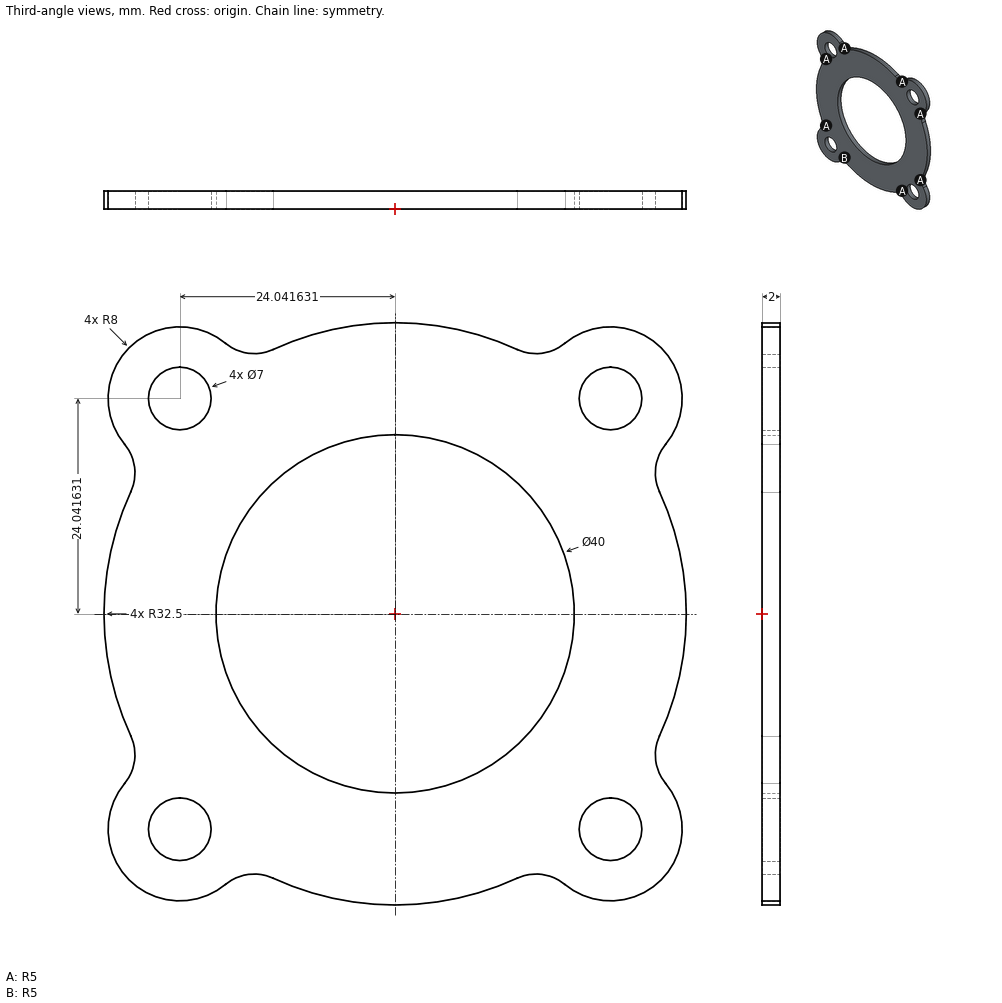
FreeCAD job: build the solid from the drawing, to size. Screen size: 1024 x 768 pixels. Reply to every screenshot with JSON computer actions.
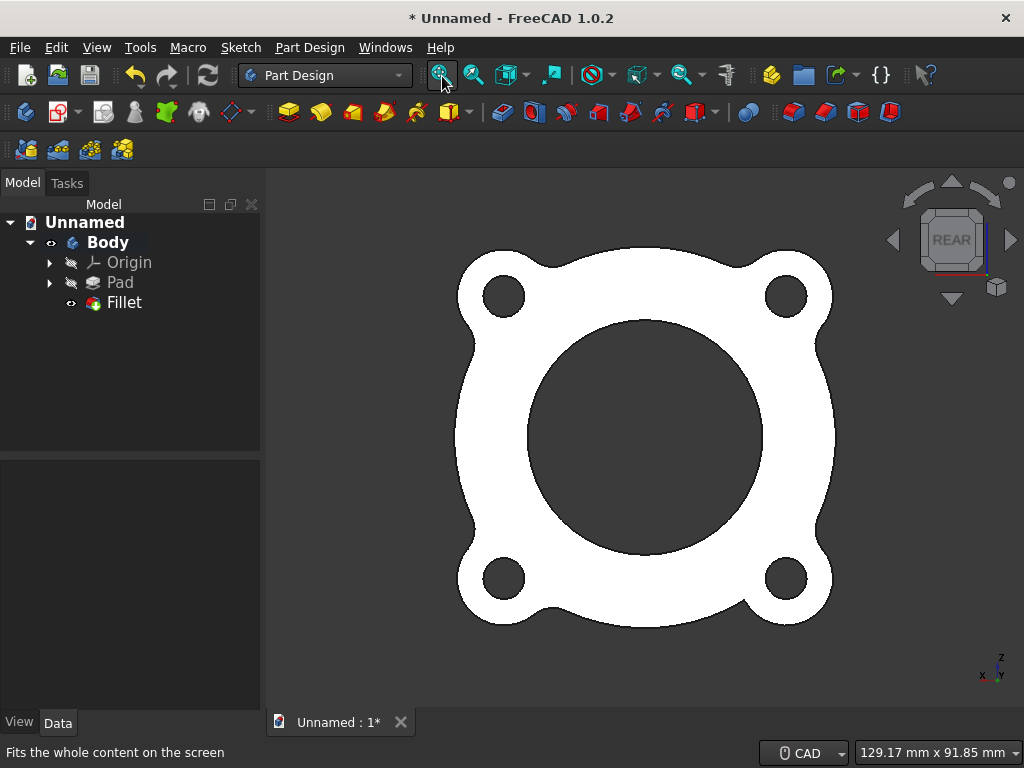
{"action": "scroll", "coordinate": [744, 599], "scroll_direction": "up", "scroll_amount": 7}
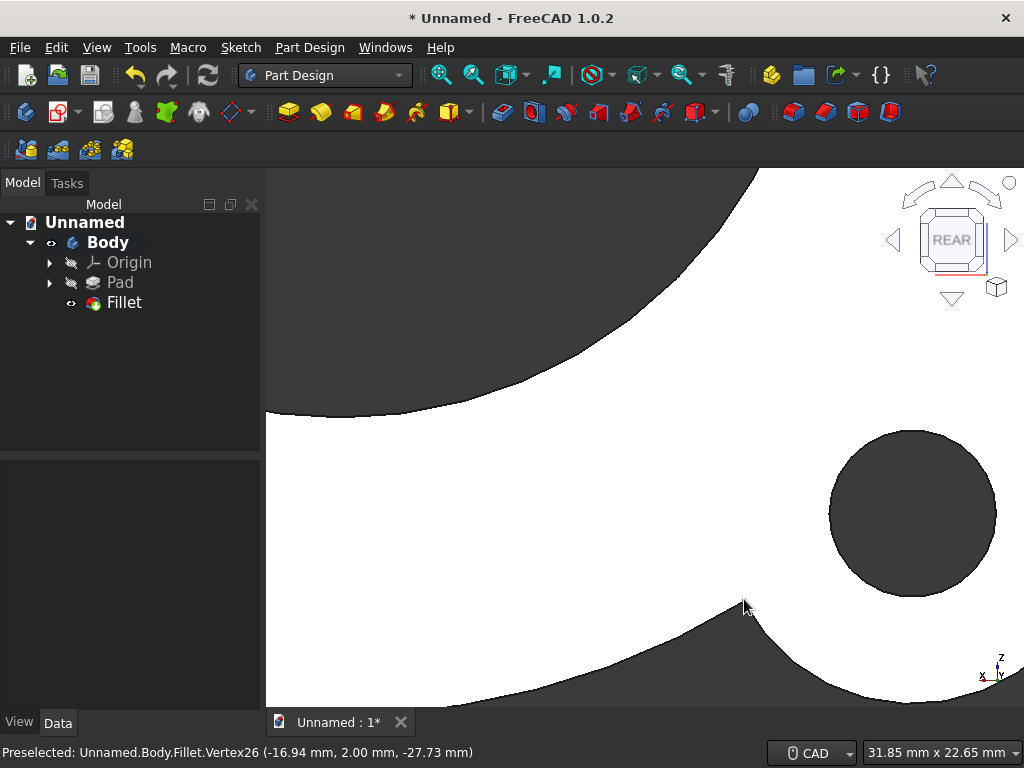
{"action": "left_click", "coordinate": [442, 76]}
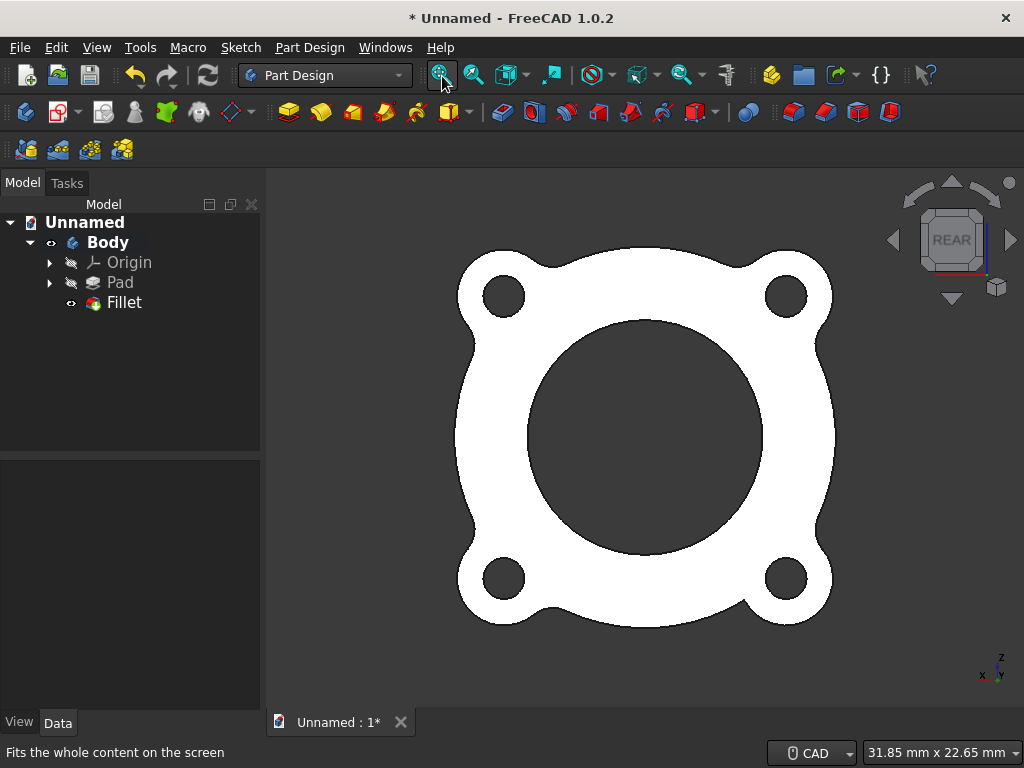
{"action": "key", "text": "6"}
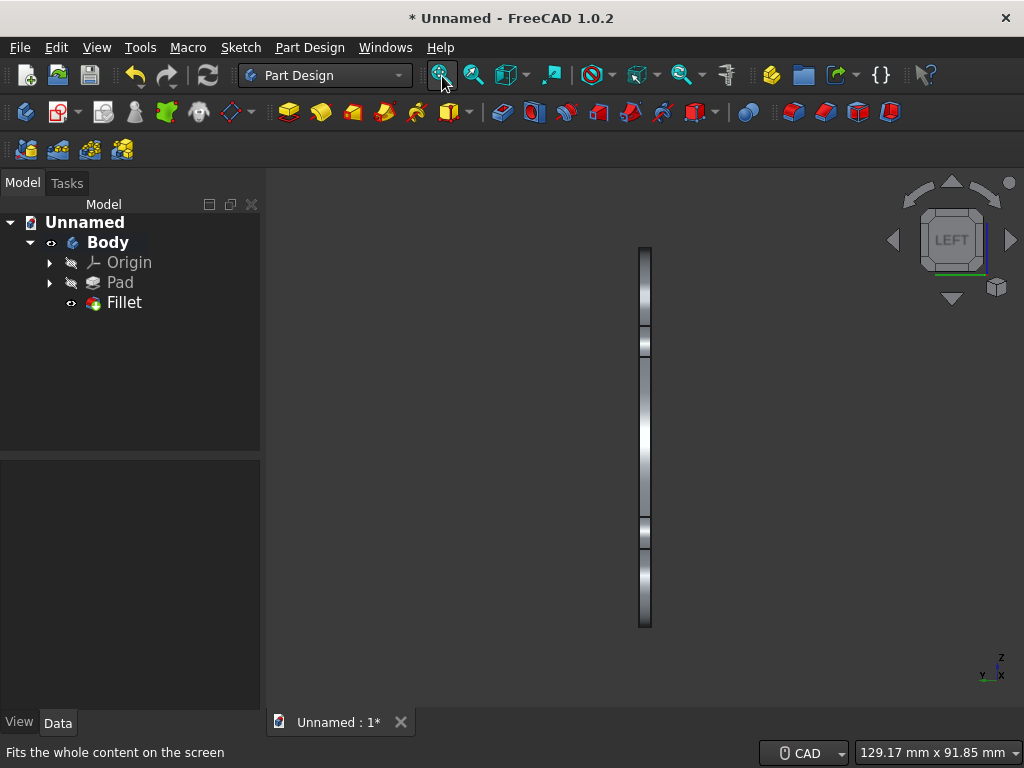
{"action": "scroll", "coordinate": [645, 599], "scroll_direction": "up", "scroll_amount": 7}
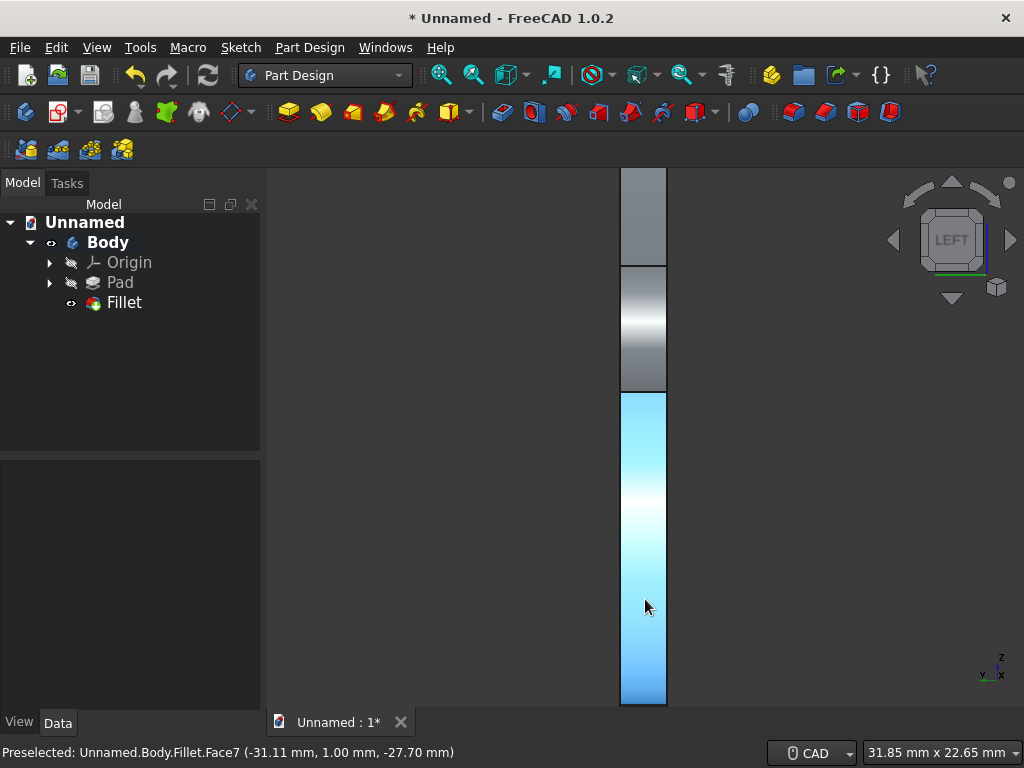
{"action": "key", "text": "v f"}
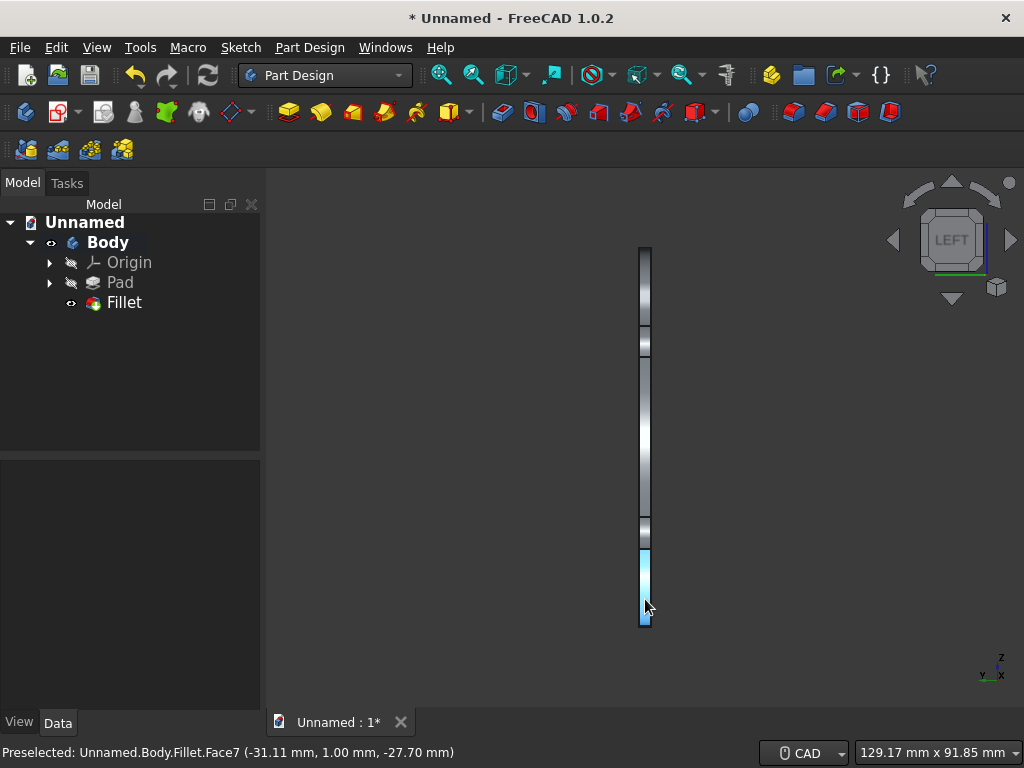
{"action": "key", "text": "v 3"}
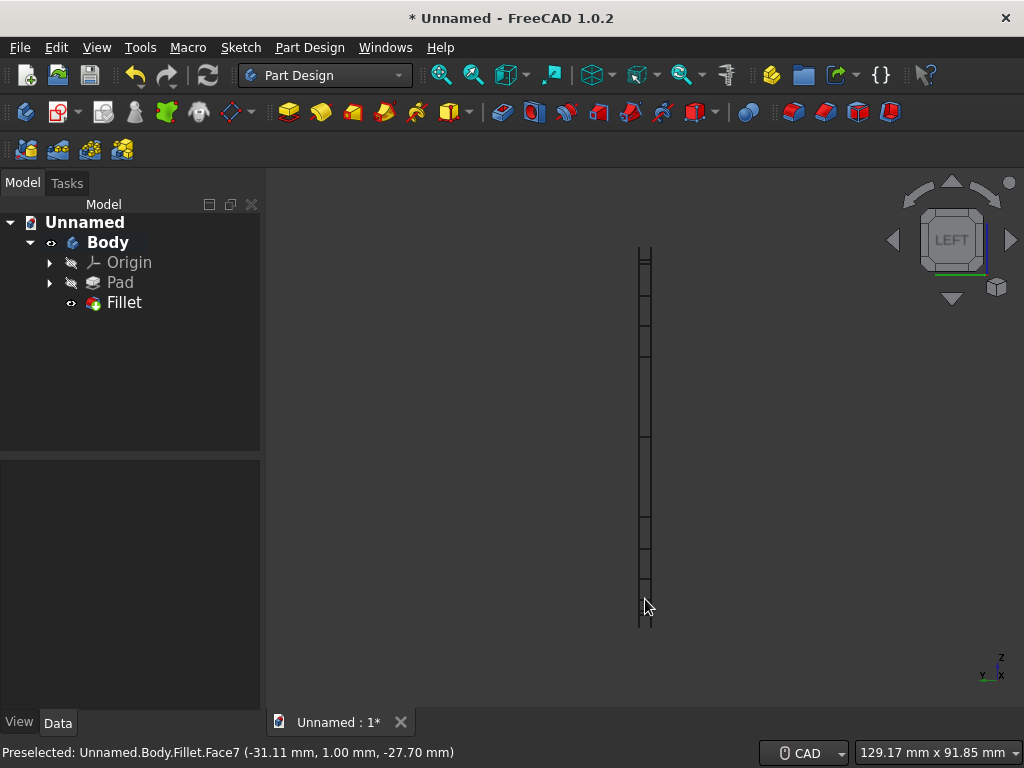
{"action": "key", "text": "0"}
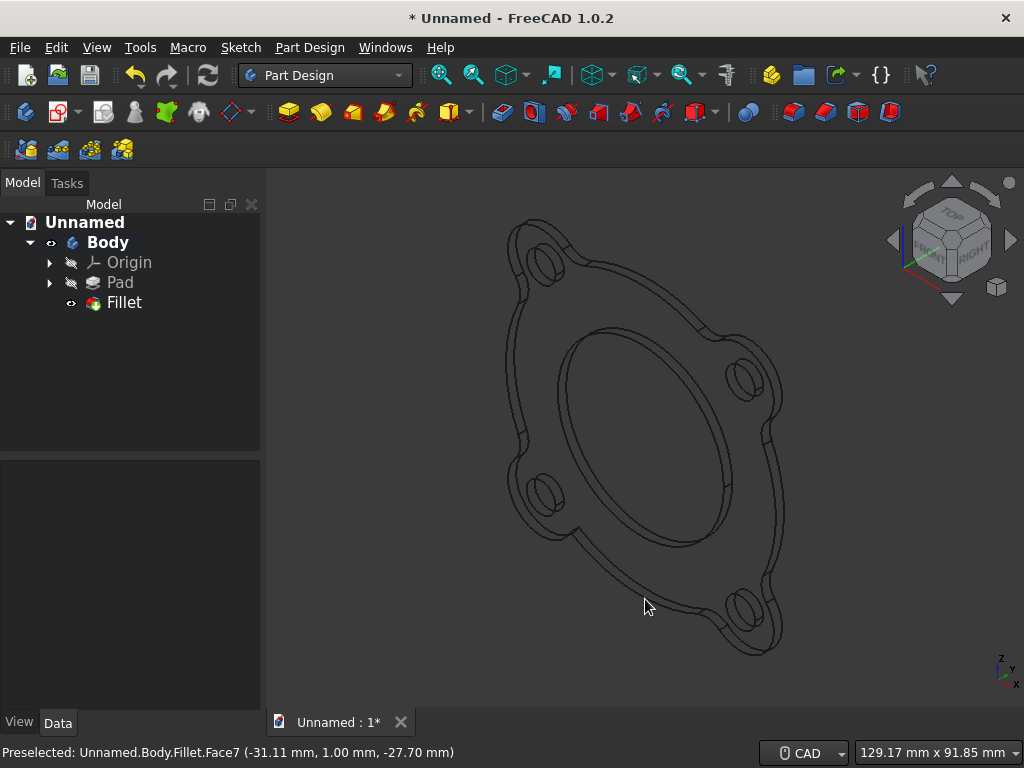
{"action": "scroll", "coordinate": [575, 529], "scroll_direction": "up", "scroll_amount": 7}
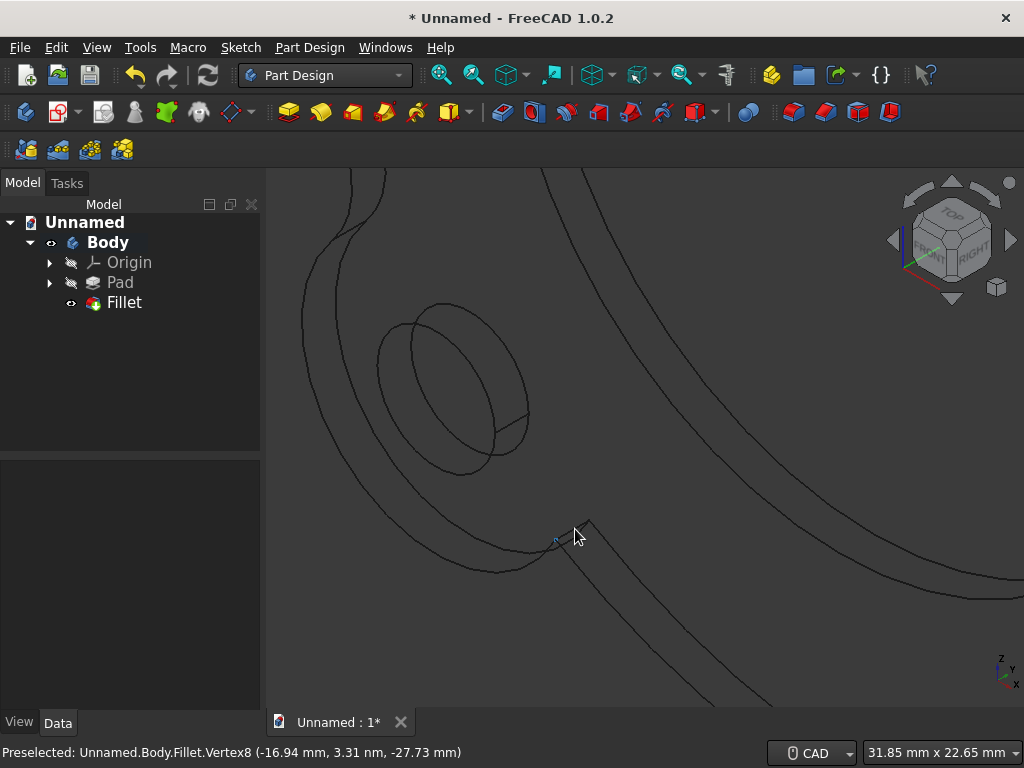
{"action": "left_click", "coordinate": [572, 529]}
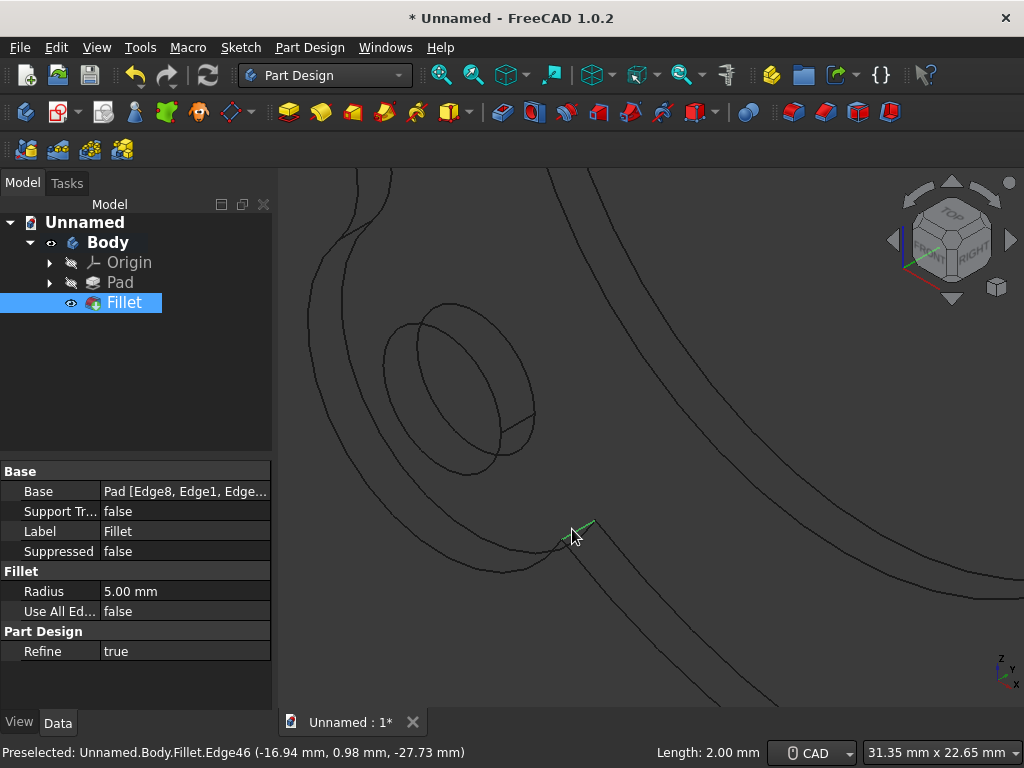
{"action": "key", "text": "v 1"}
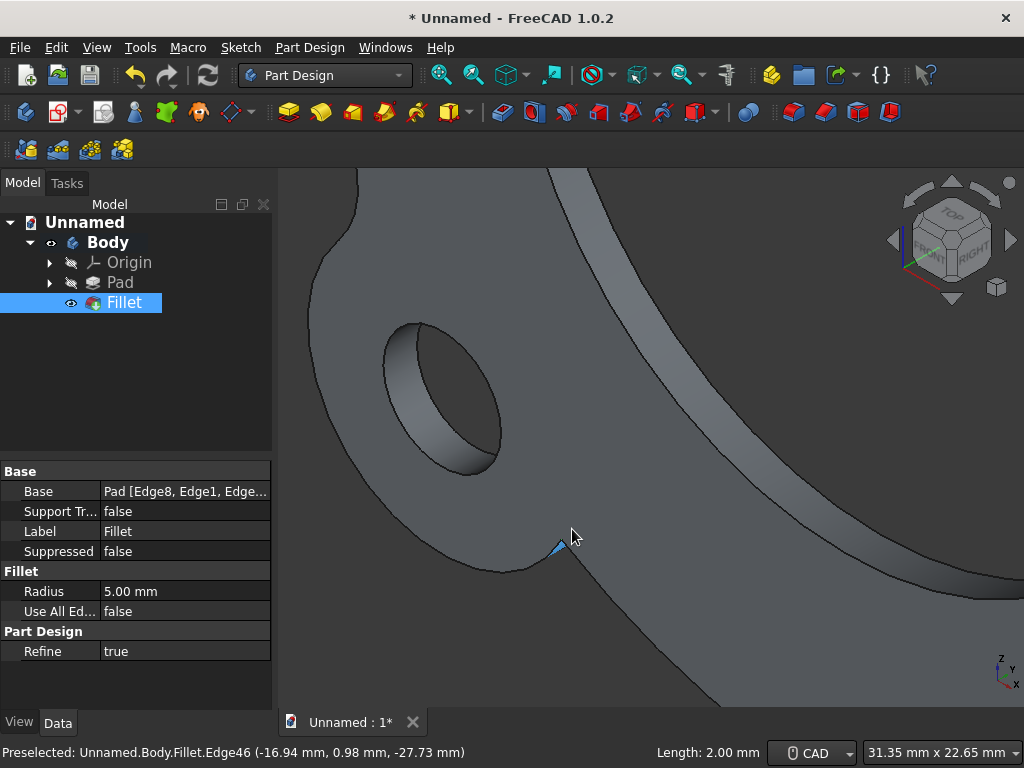
{"action": "left_click", "coordinate": [794, 112]}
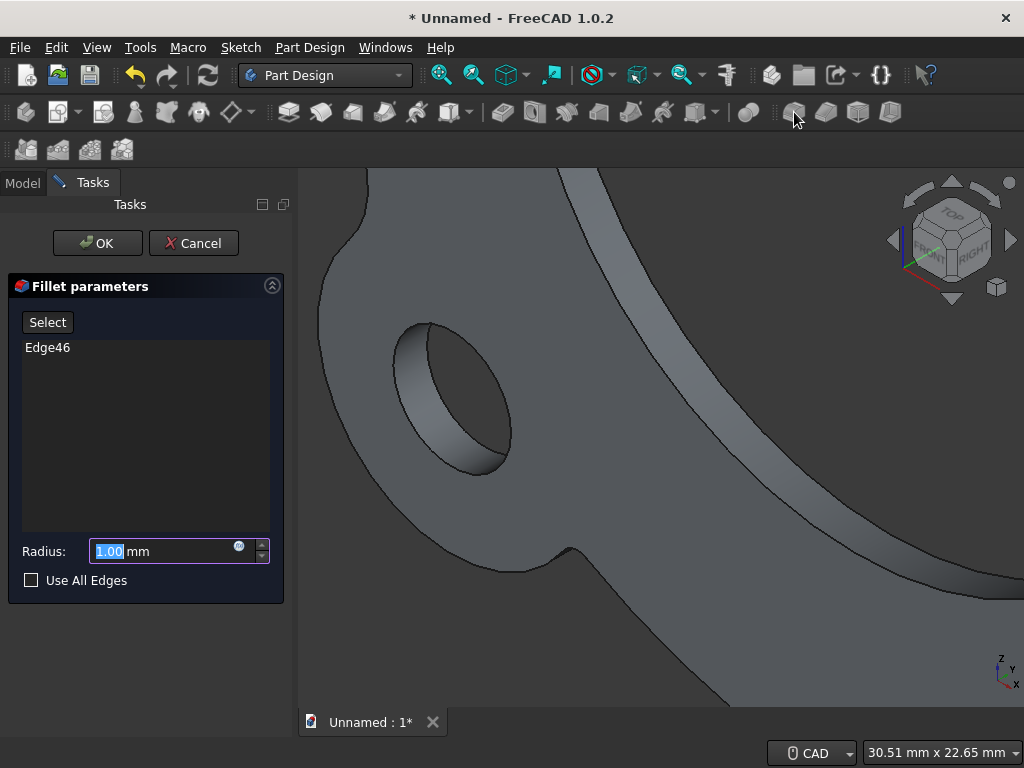
{"action": "type", "text": "5"}
{"action": "key", "text": "Tab"}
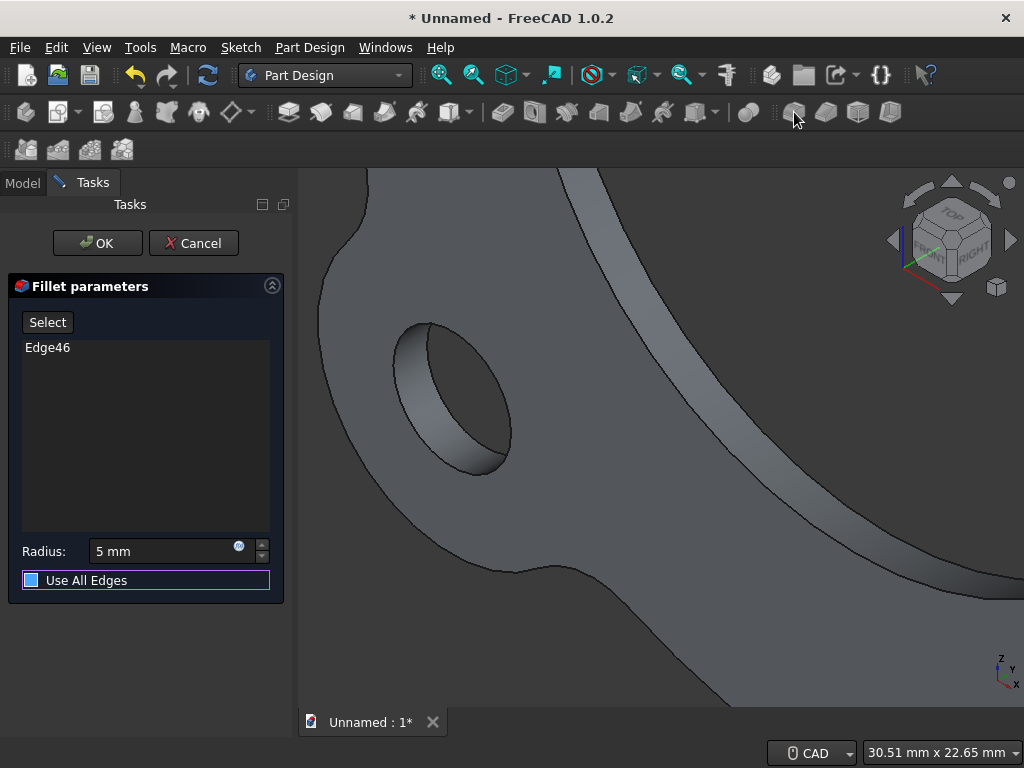
{"action": "left_click", "coordinate": [98, 243]}